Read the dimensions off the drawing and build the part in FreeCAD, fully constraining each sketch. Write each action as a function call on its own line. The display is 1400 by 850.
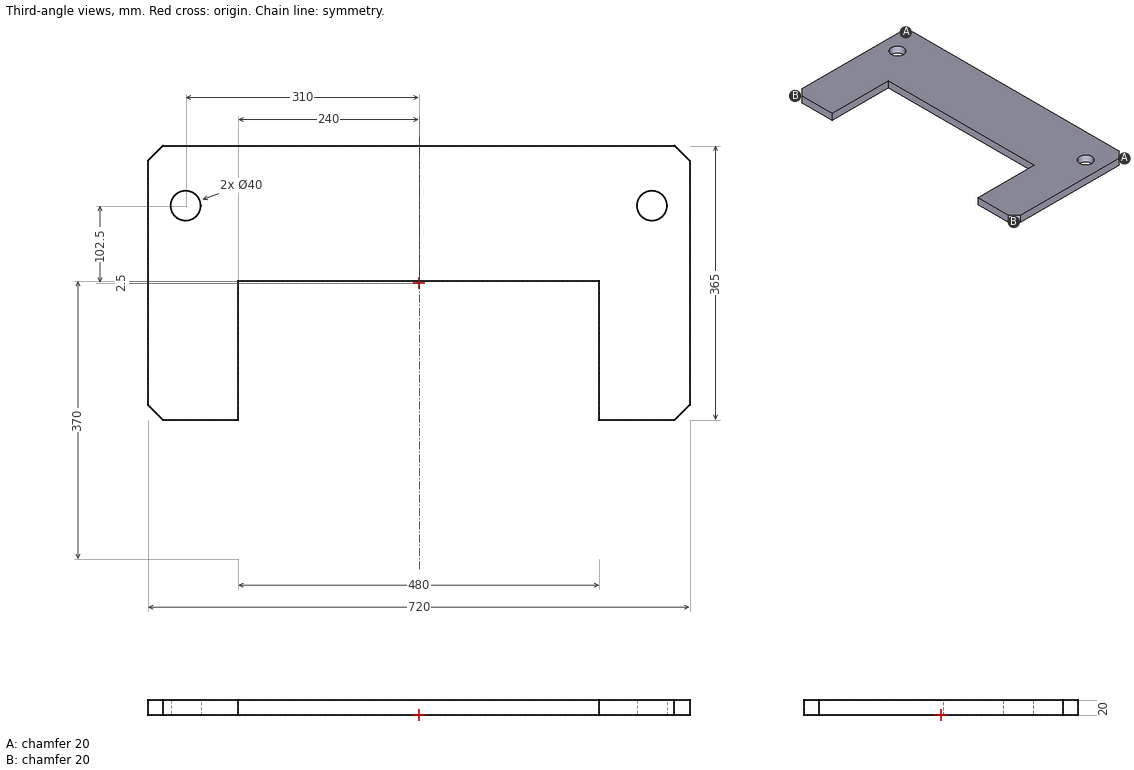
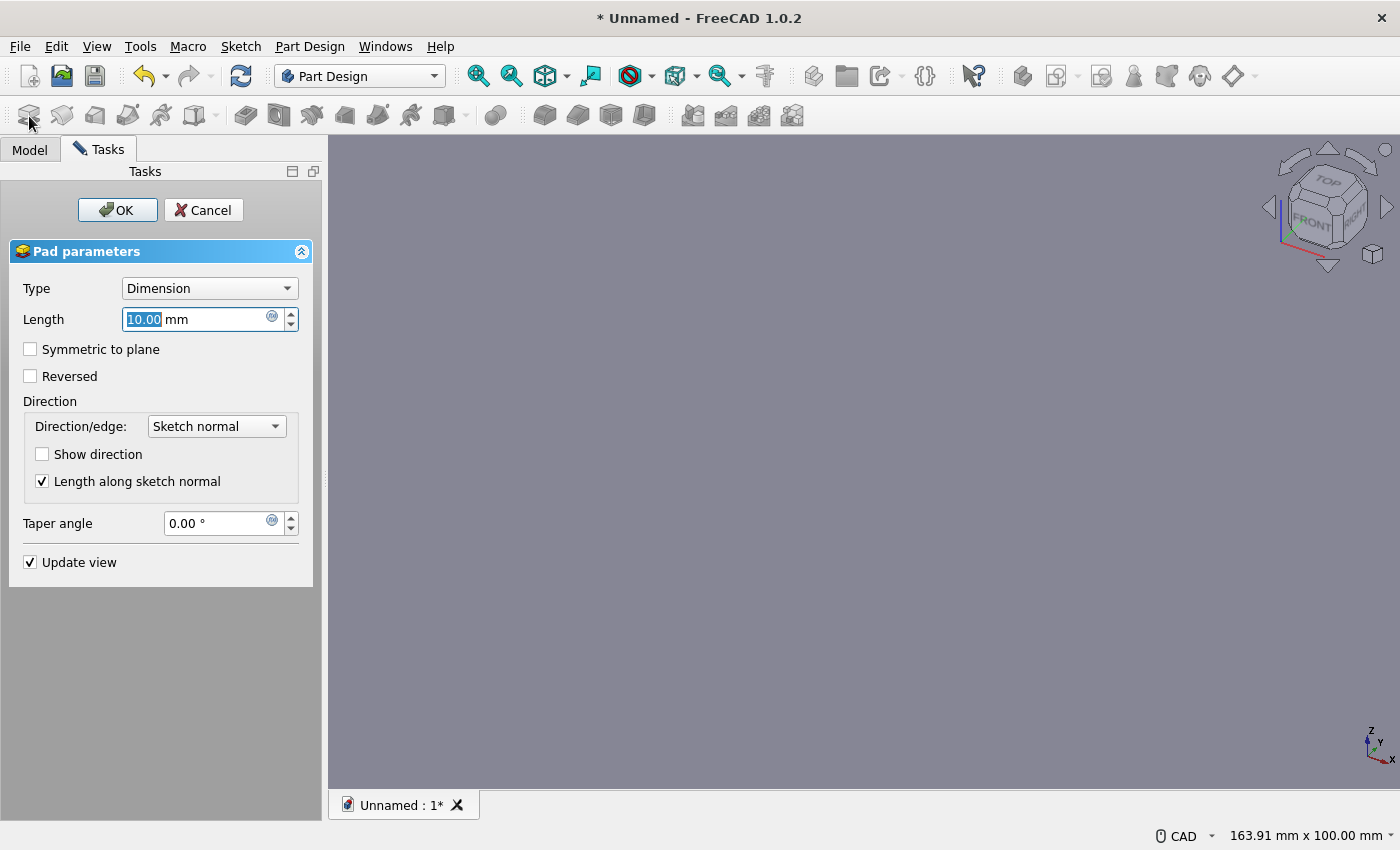
text(20)
key(Tab)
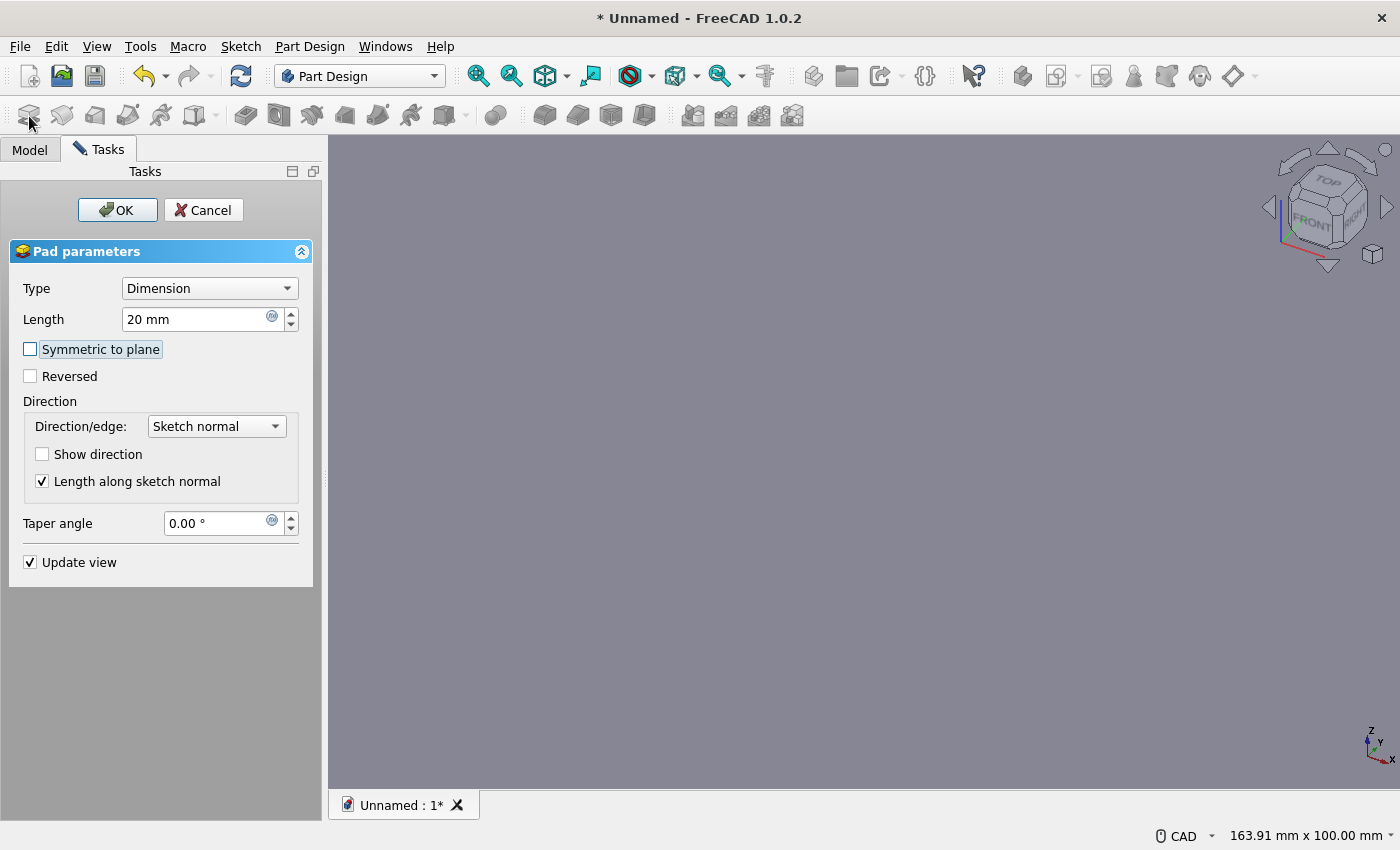
click(118, 210)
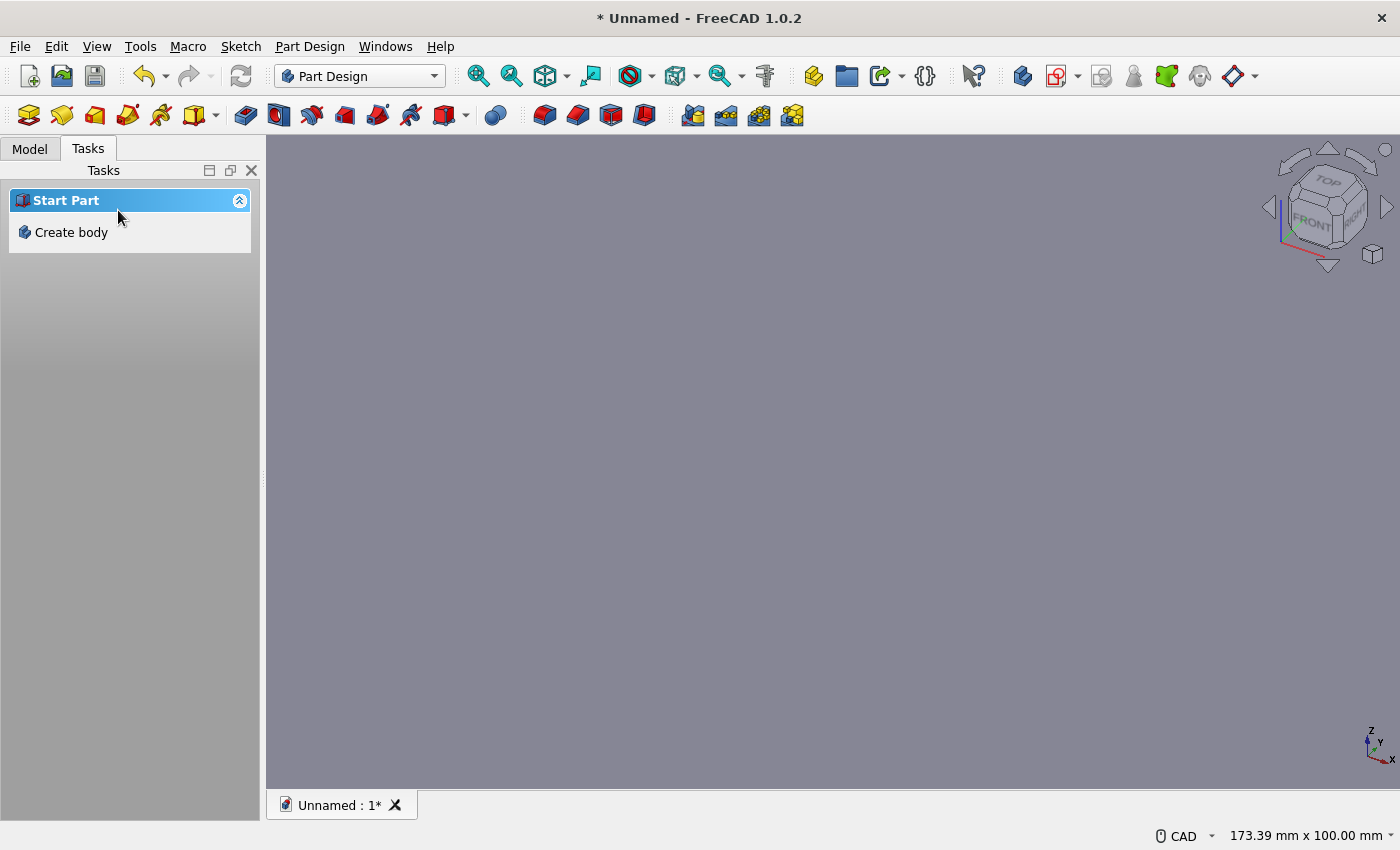
key(v)
key(f)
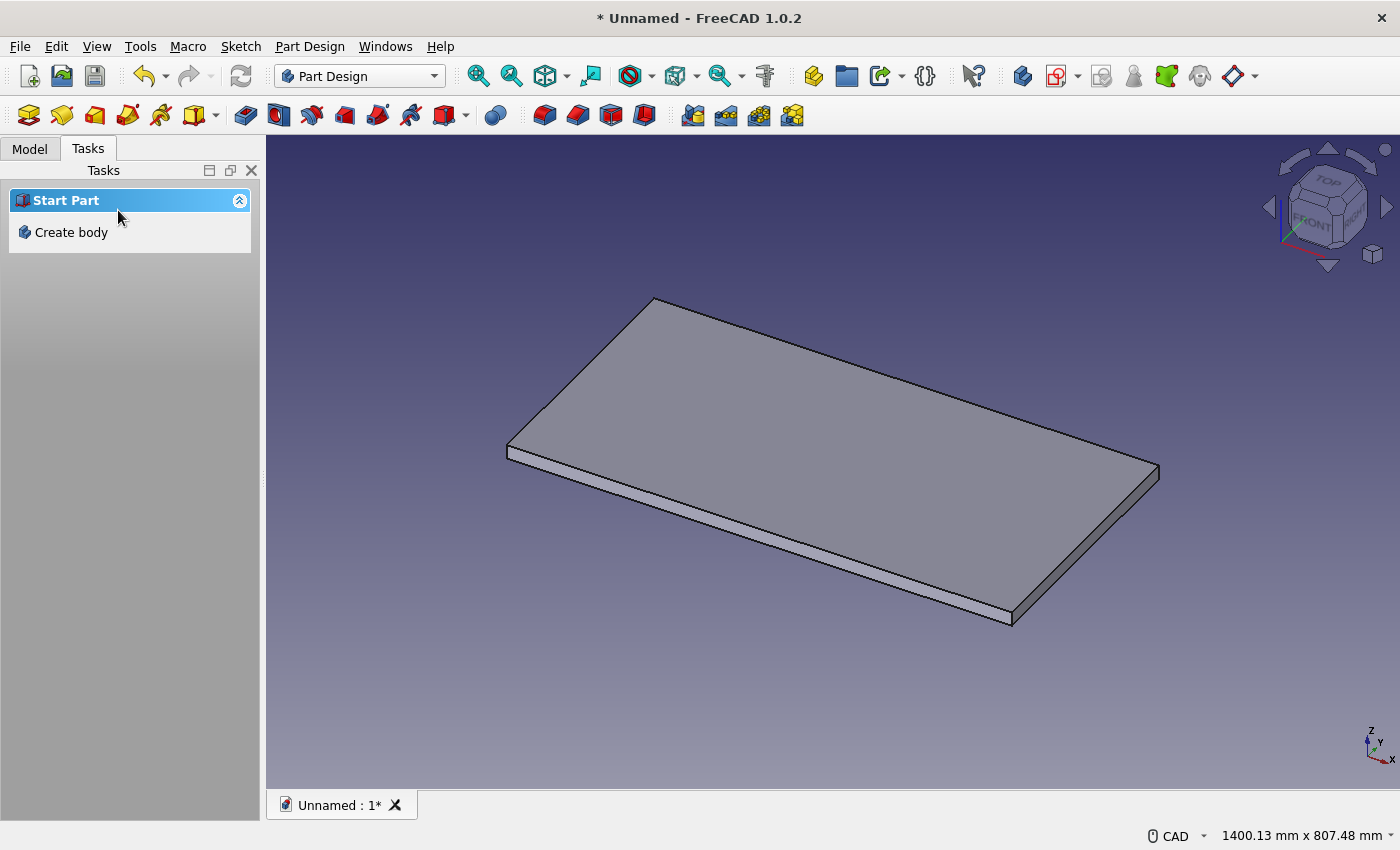
click(905, 478)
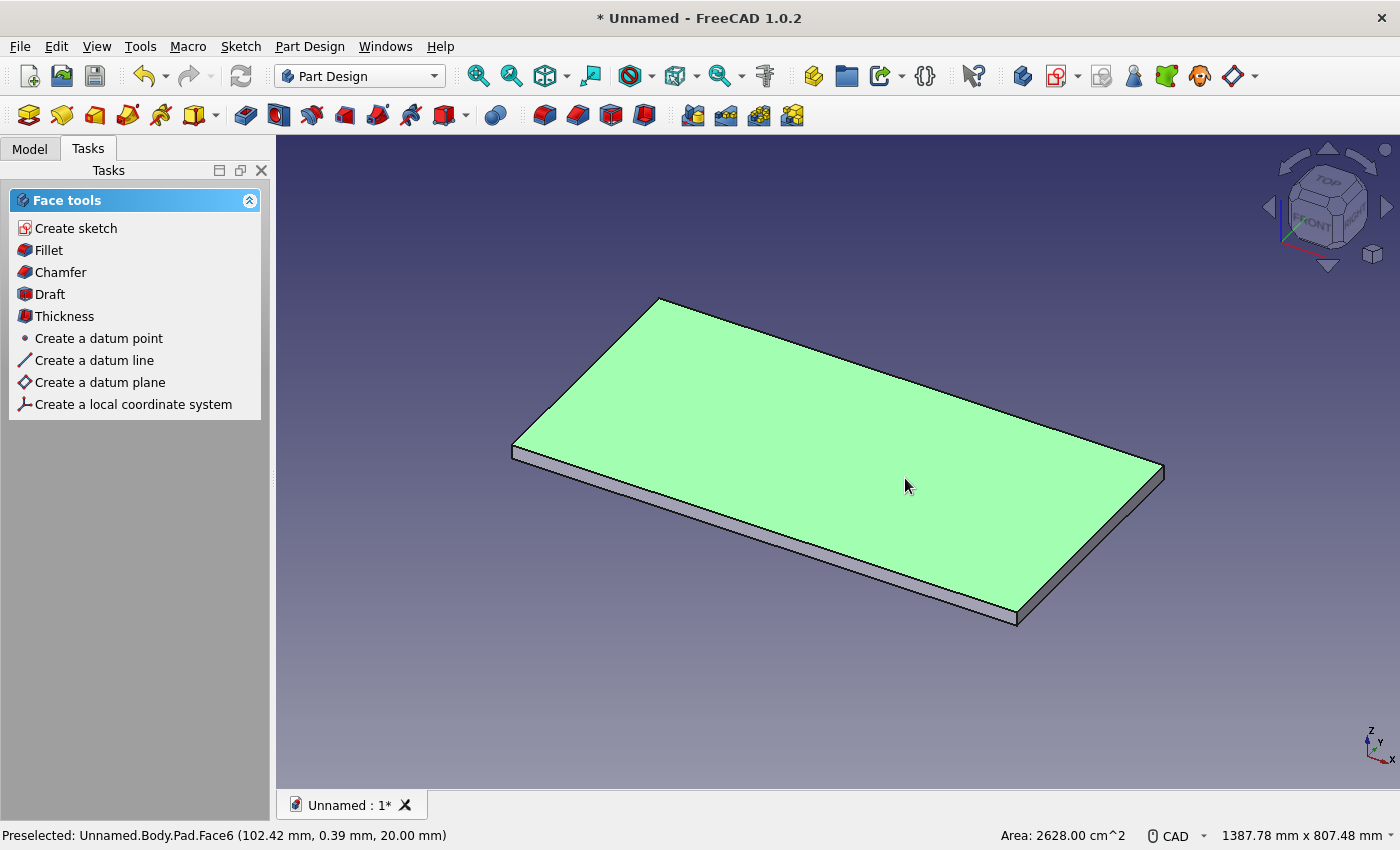
click(1056, 76)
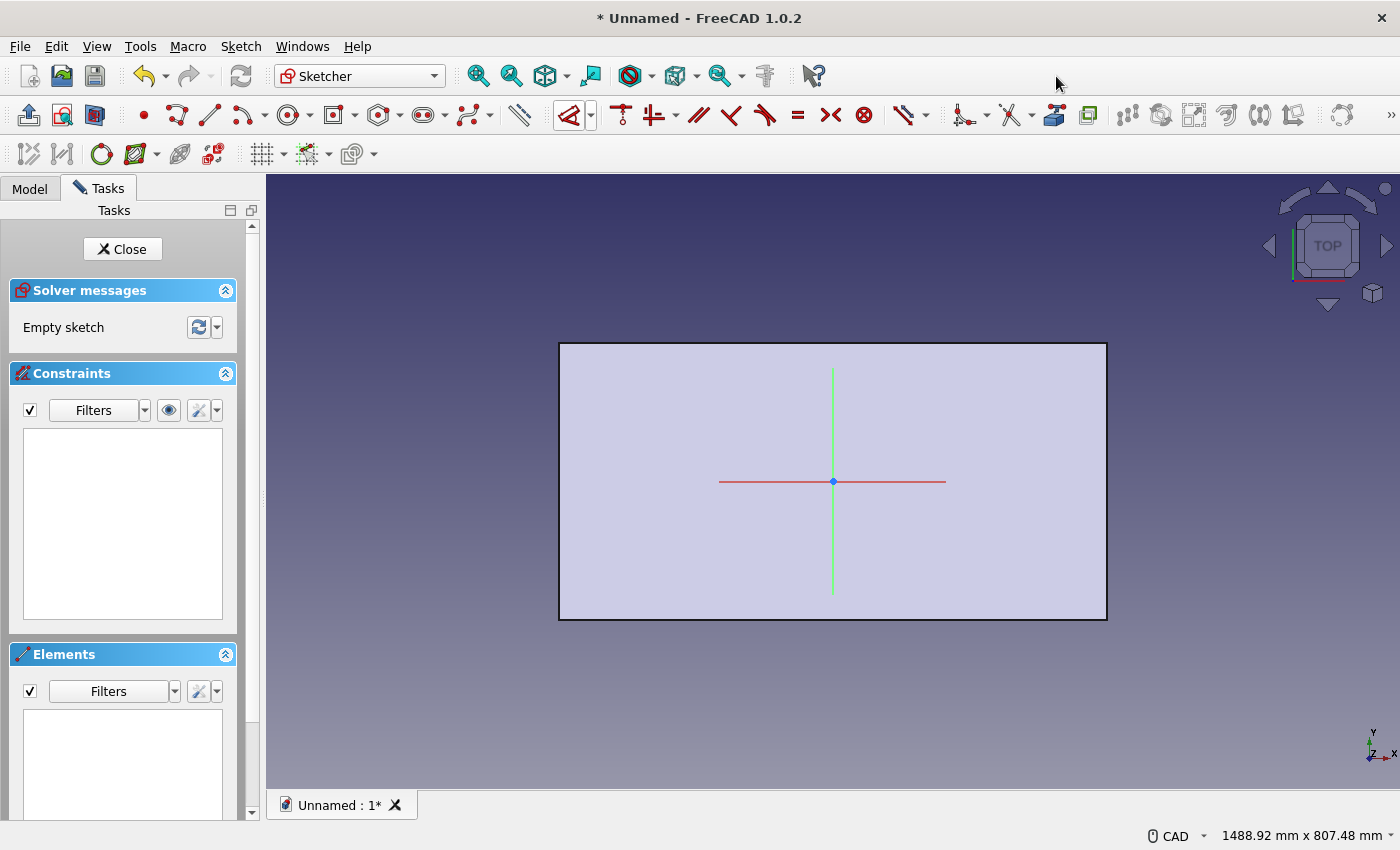
key(g)
key(c)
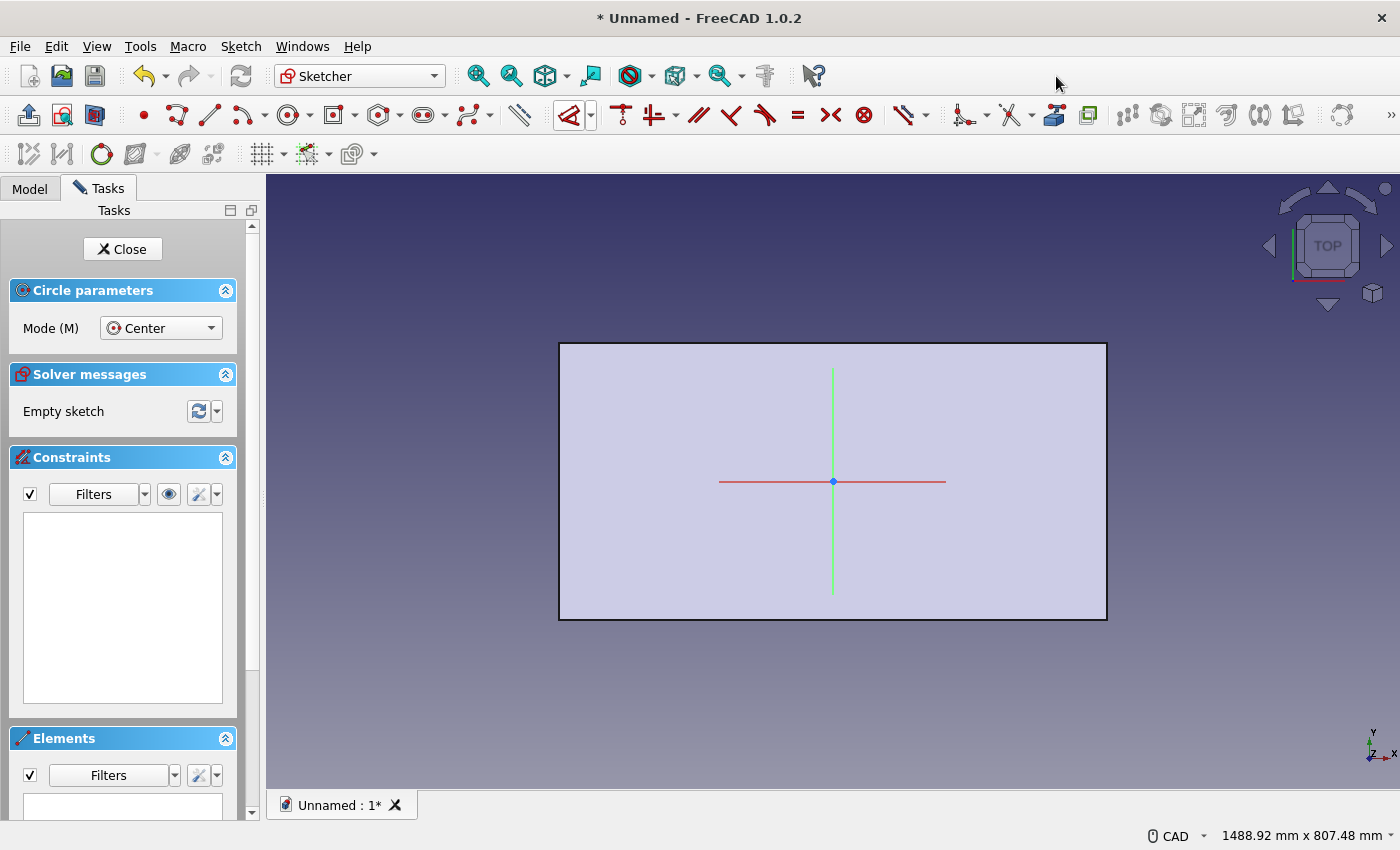
scroll(597, 403, up, 2)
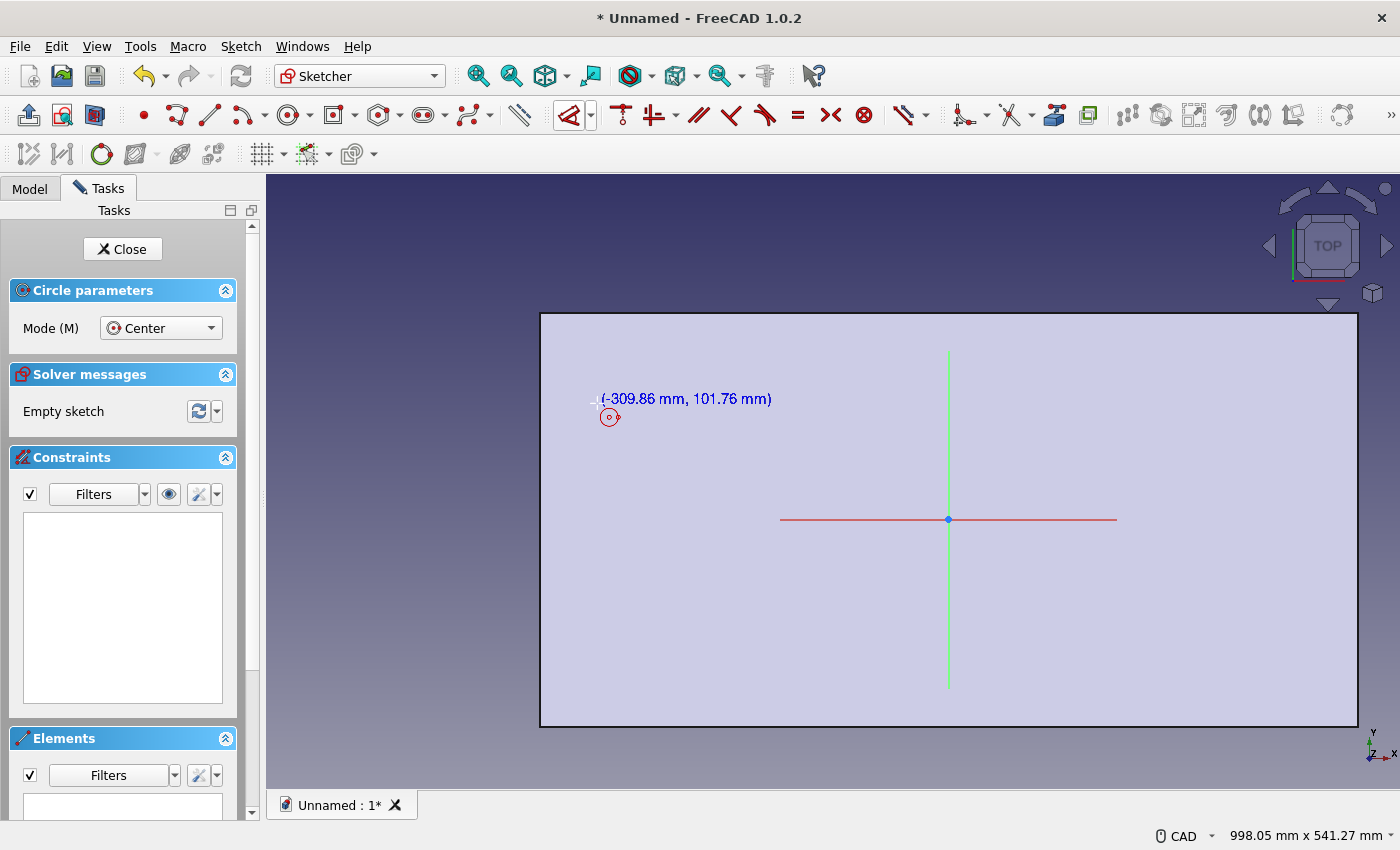
click(597, 403)
click(613, 387)